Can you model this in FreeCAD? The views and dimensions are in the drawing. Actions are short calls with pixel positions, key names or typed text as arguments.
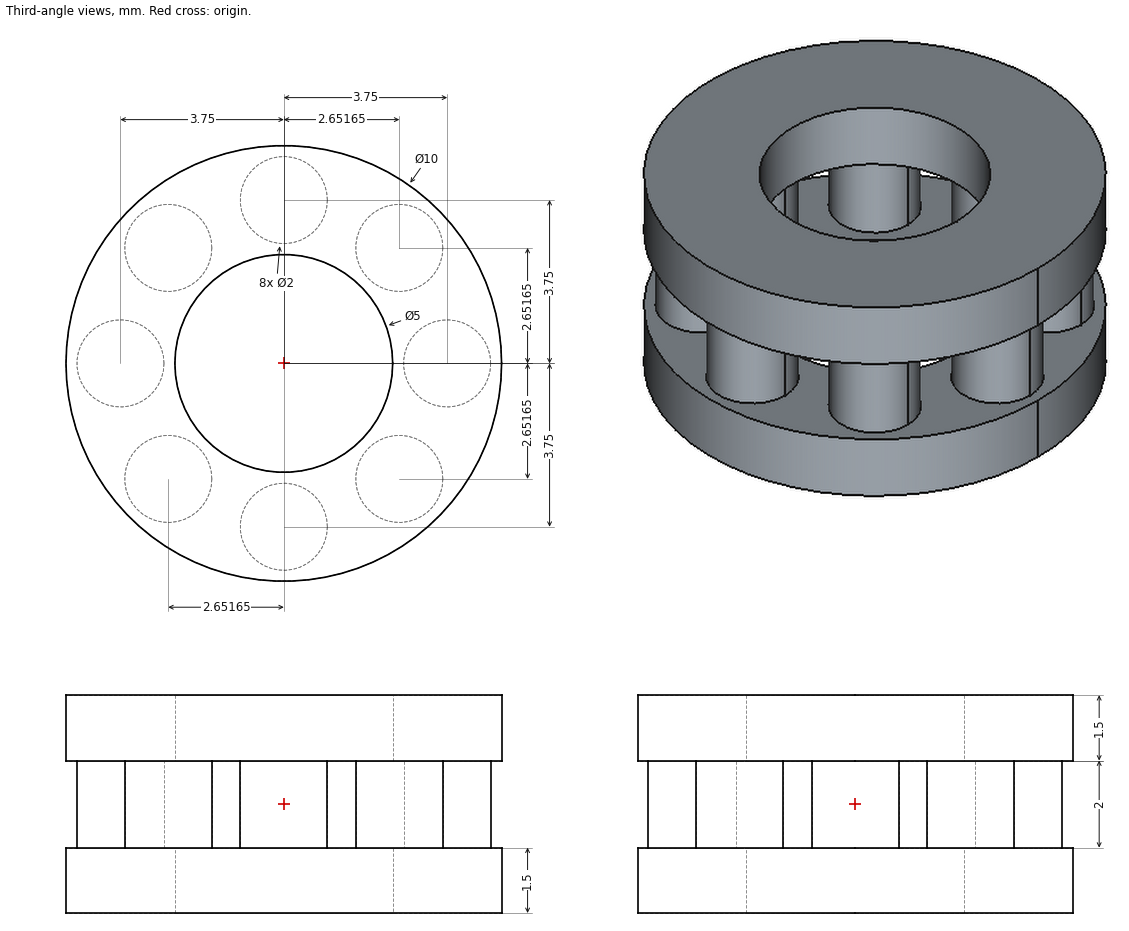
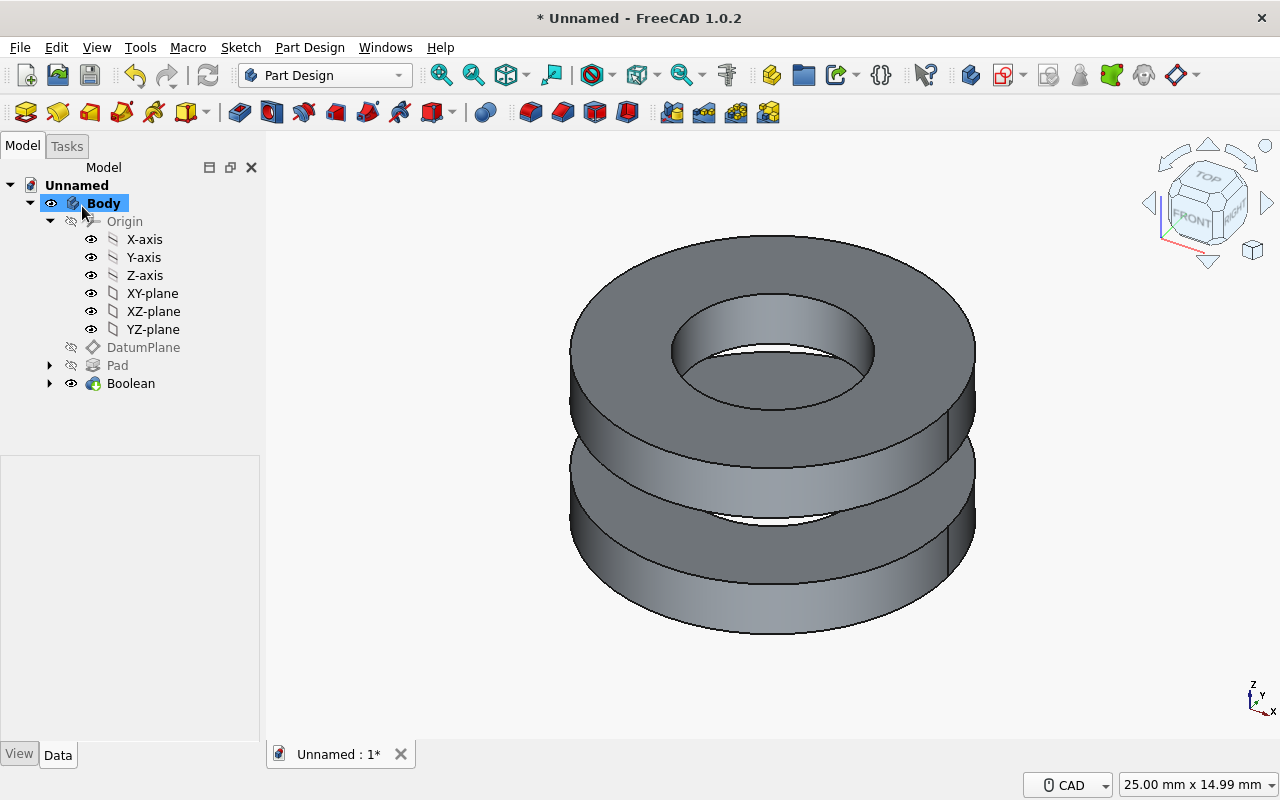
click(136, 293)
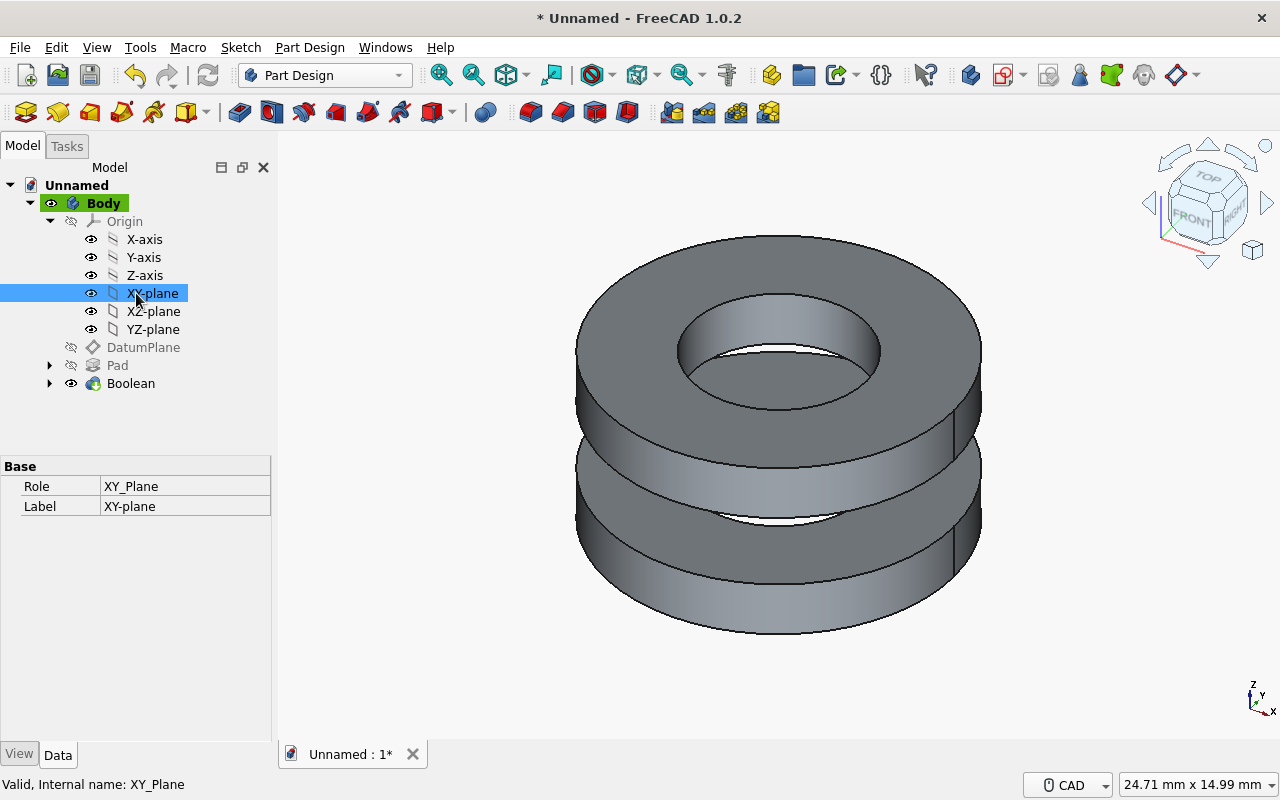
click(1176, 76)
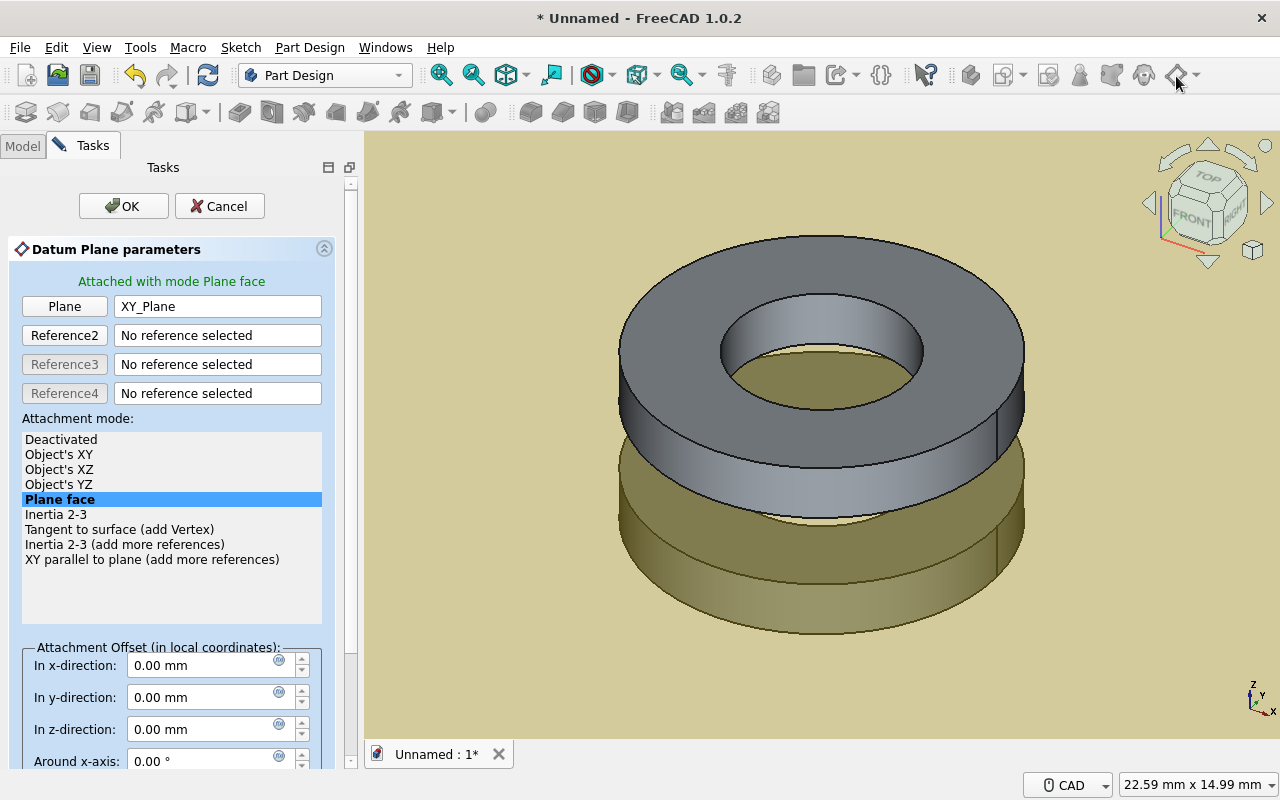
triple_click(210, 729)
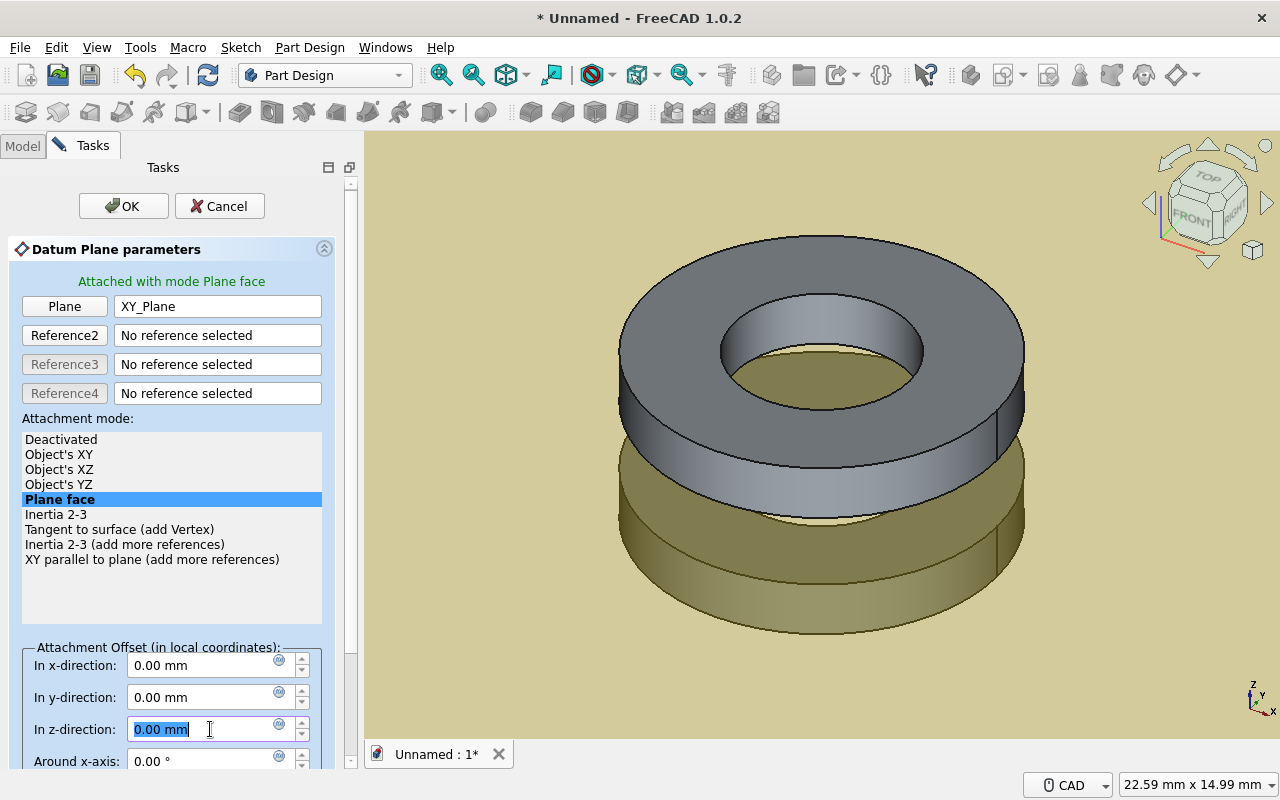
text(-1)
key(Tab)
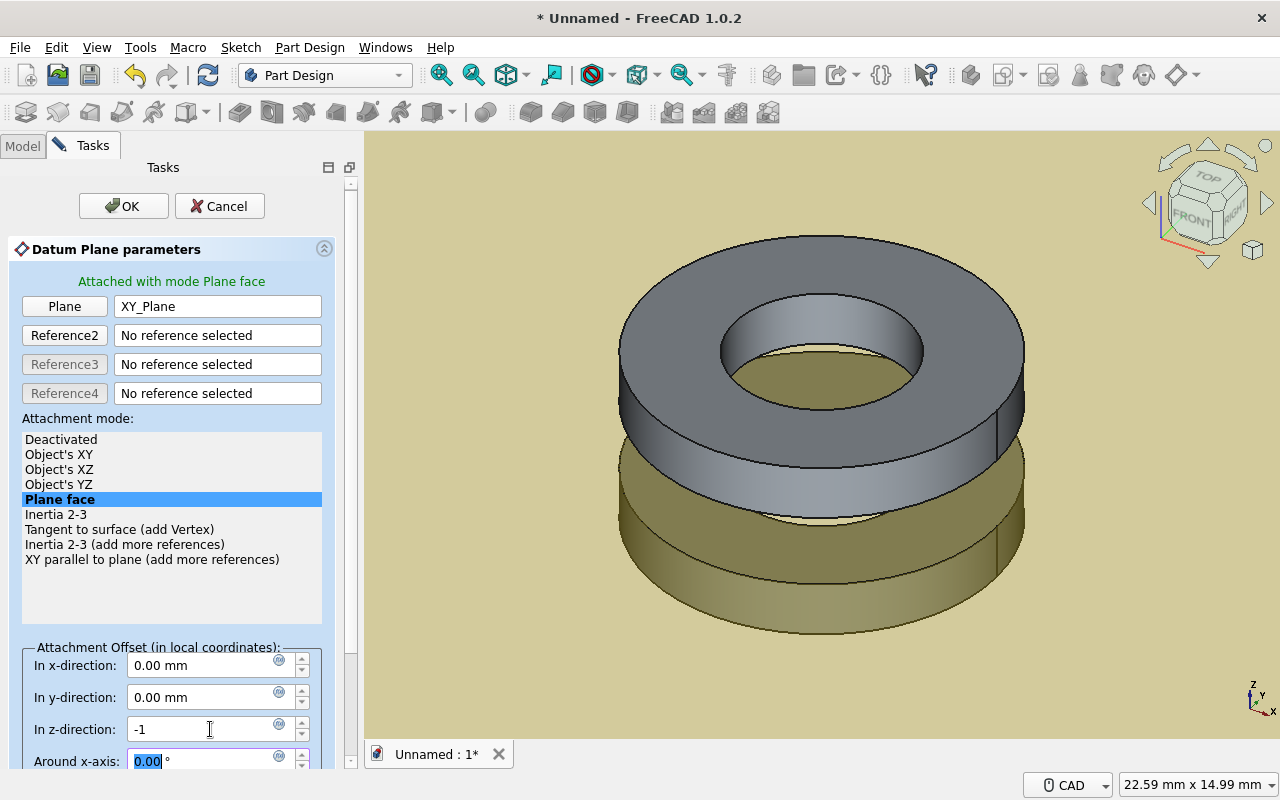
click(124, 206)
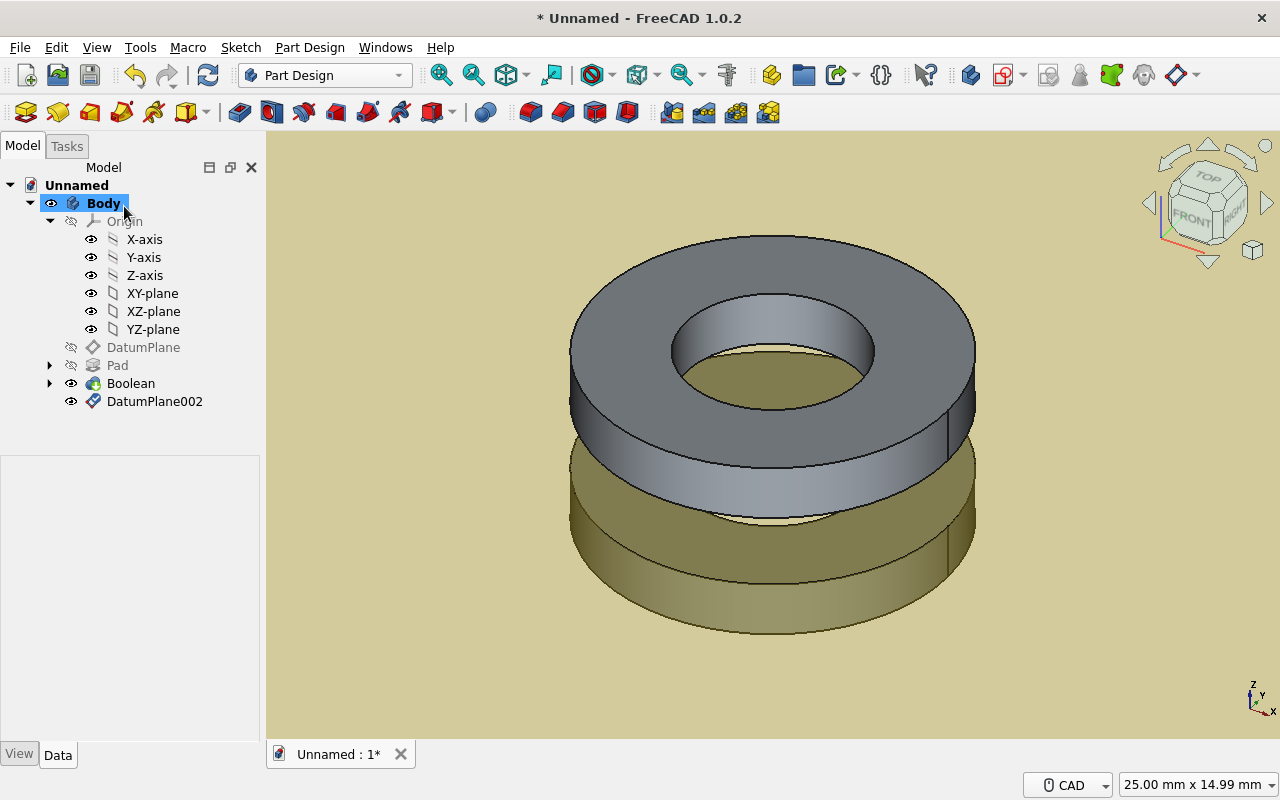
click(116, 401)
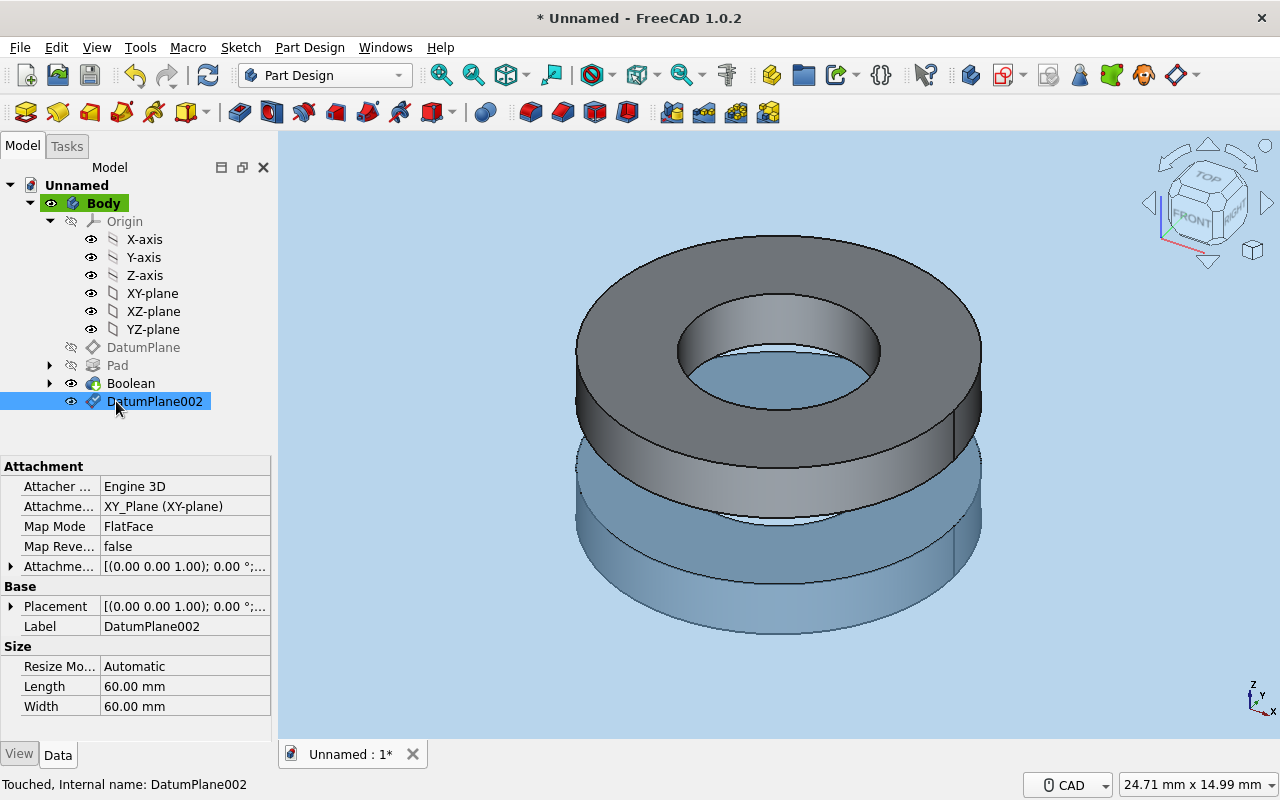
click(1004, 76)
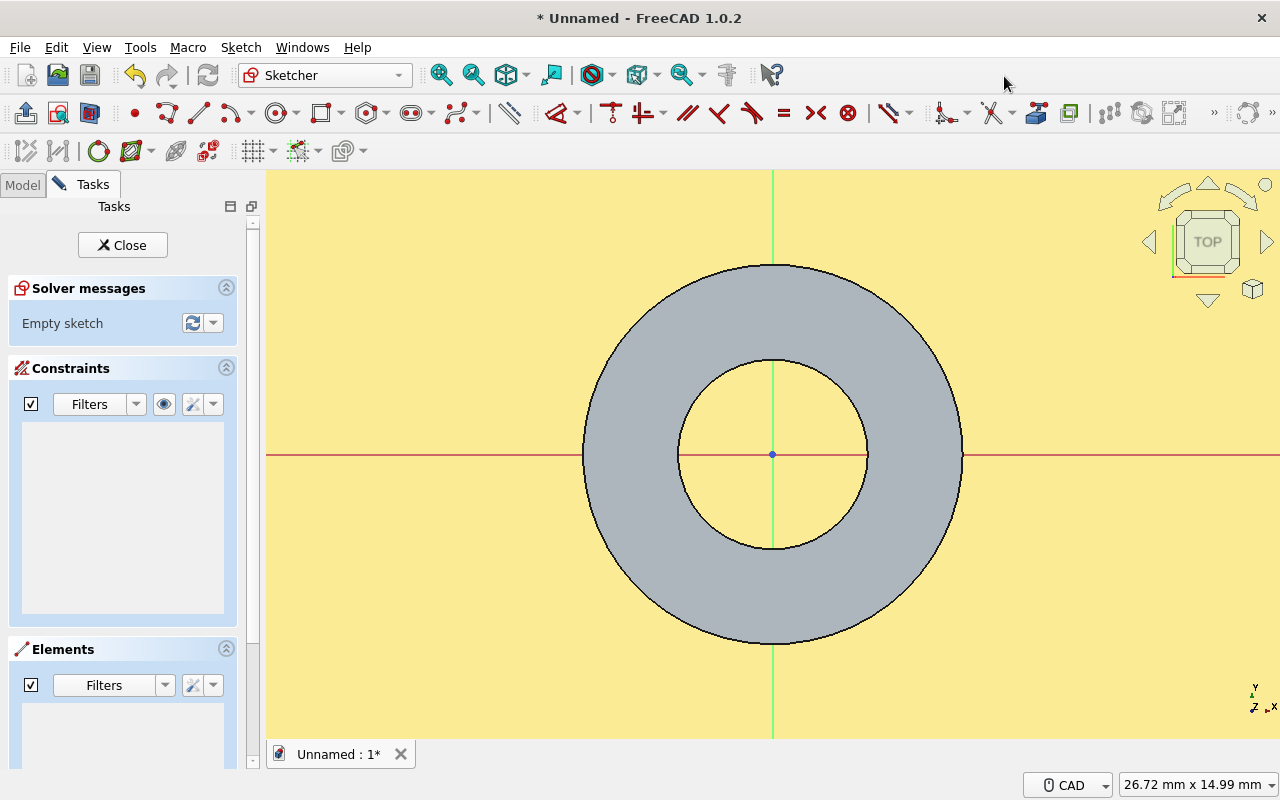
click(90, 114)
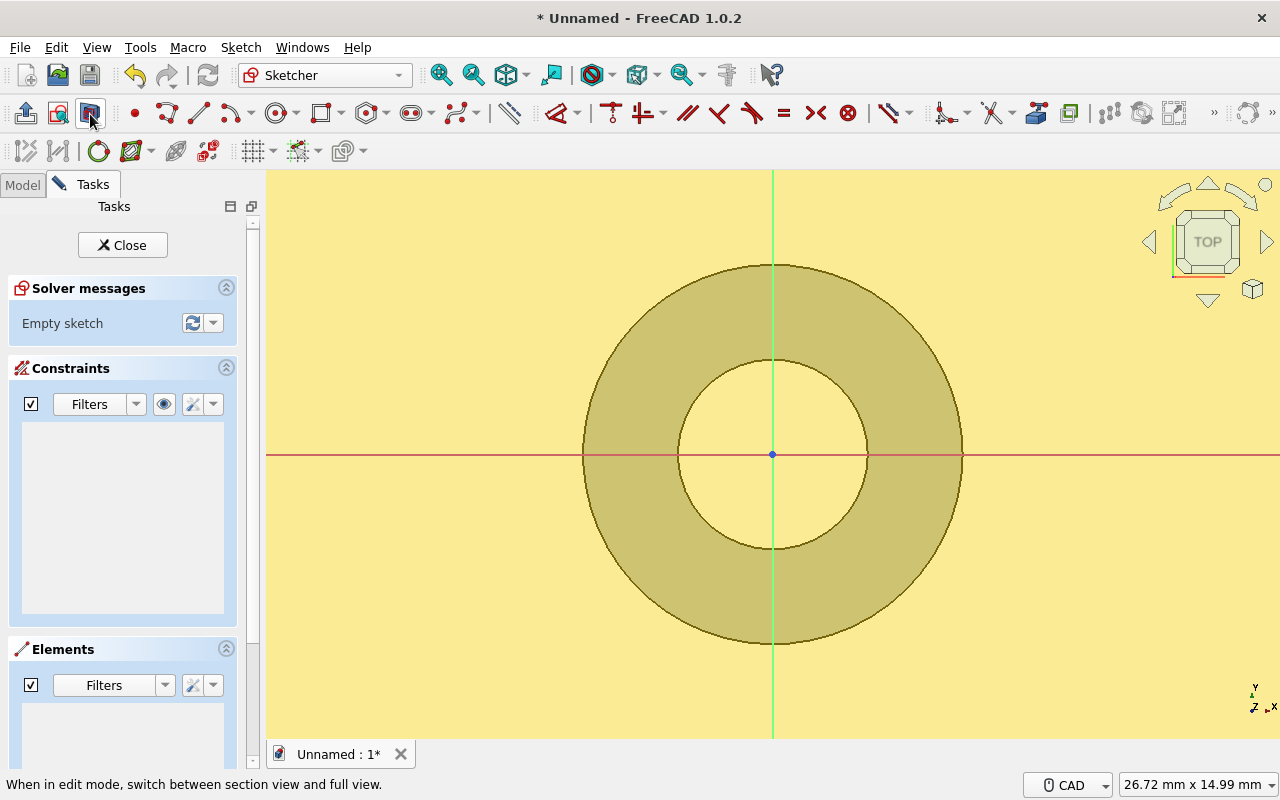
key(g)
key(c)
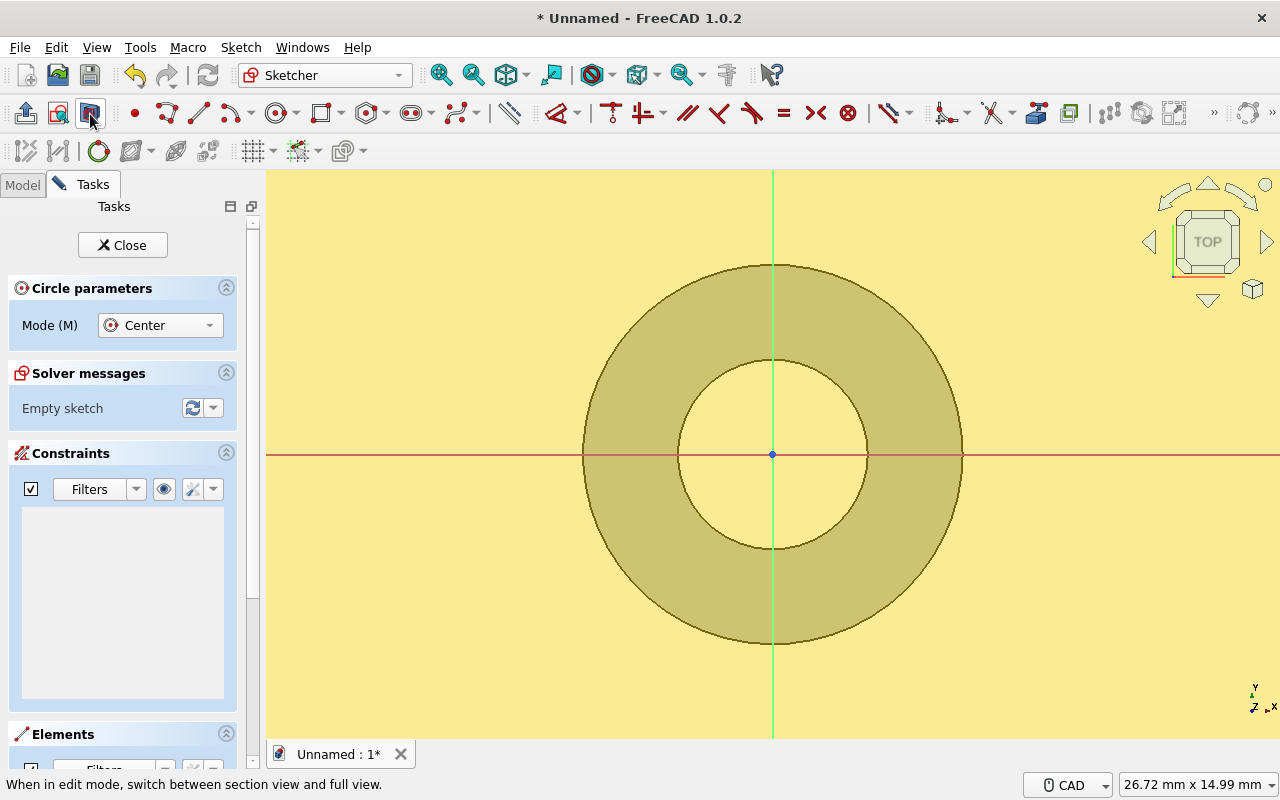
click(773, 312)
move(800, 285)